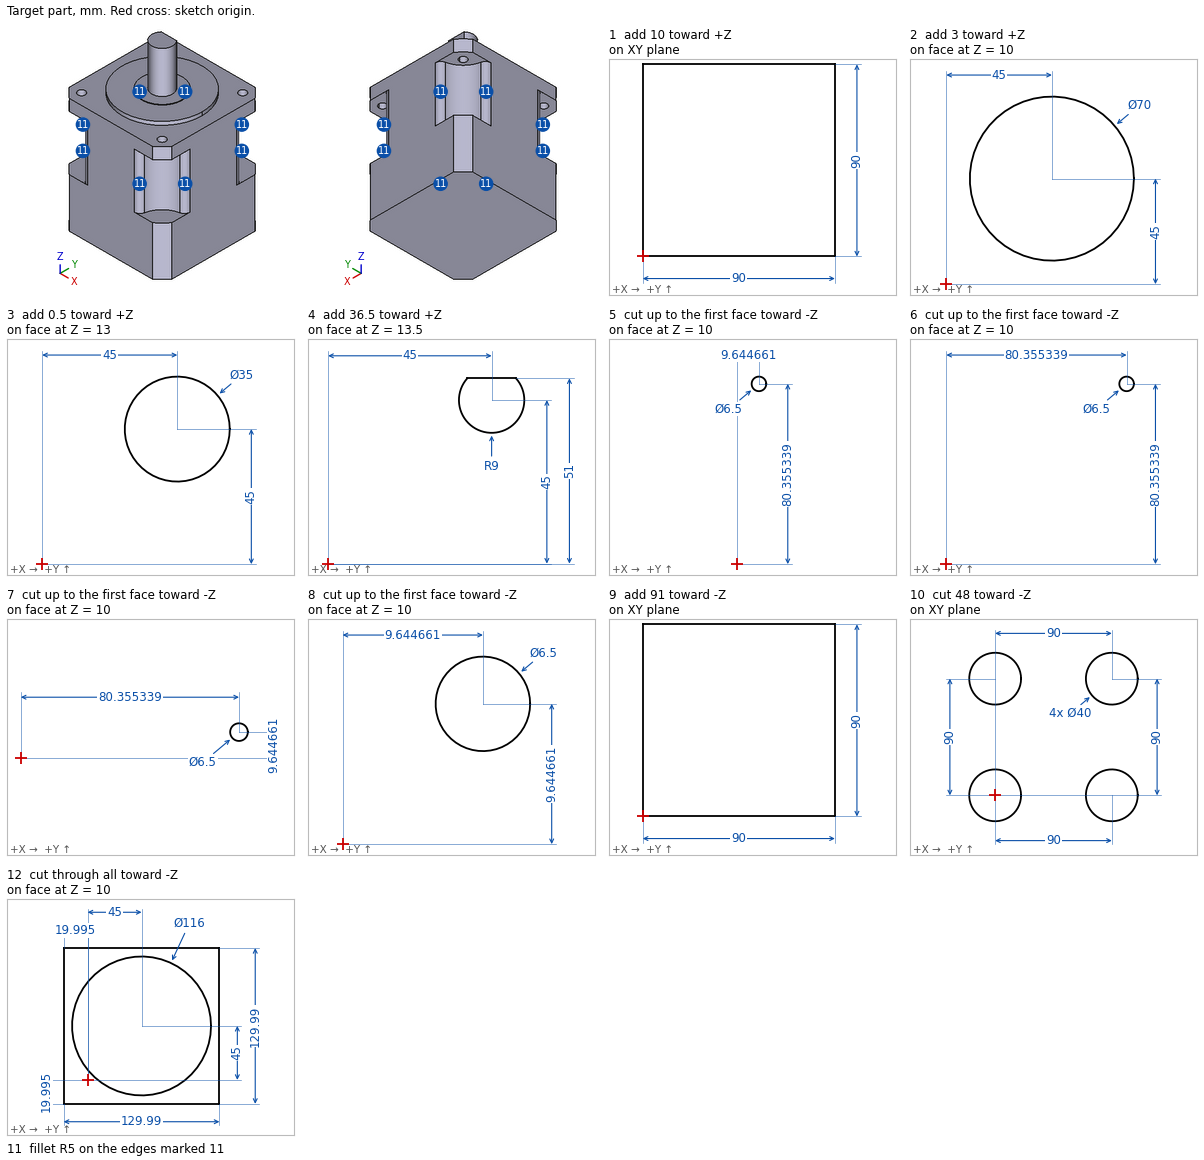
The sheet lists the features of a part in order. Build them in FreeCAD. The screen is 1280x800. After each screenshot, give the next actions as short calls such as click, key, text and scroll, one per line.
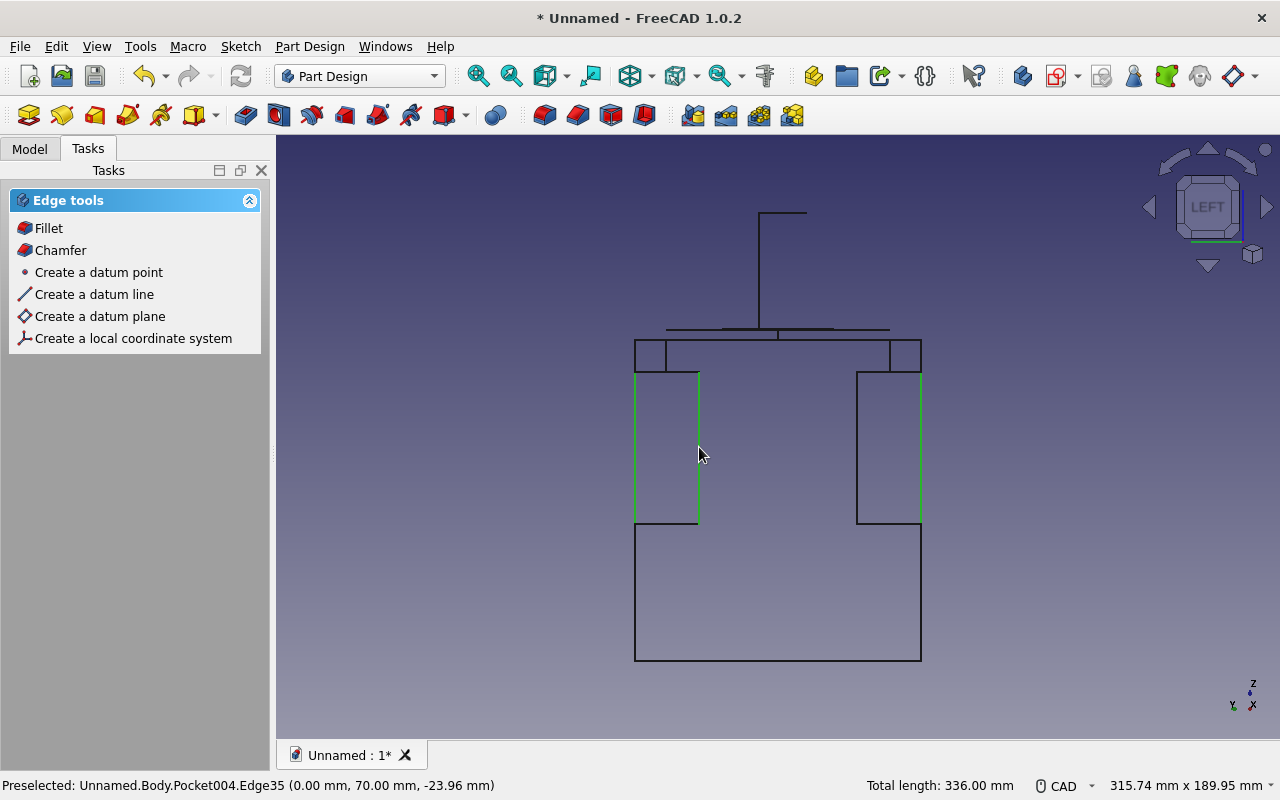
key(0)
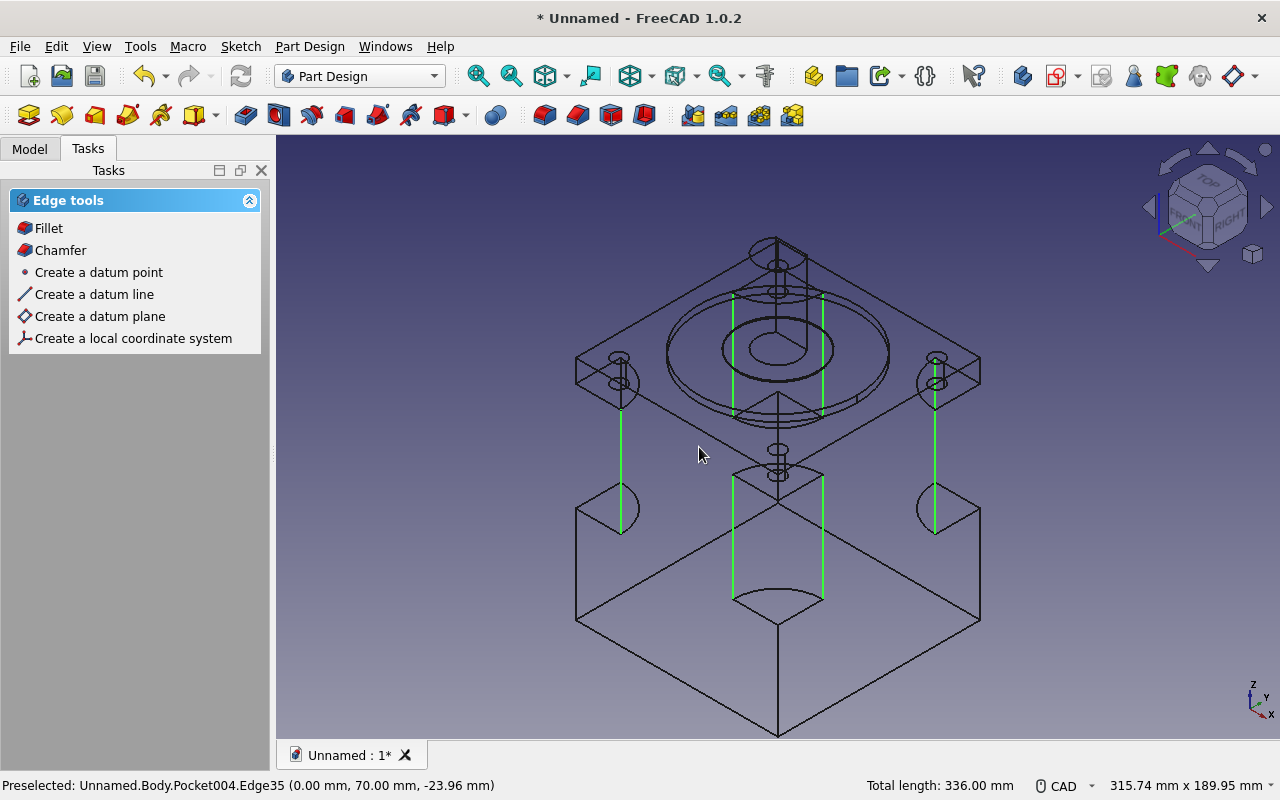
key(2)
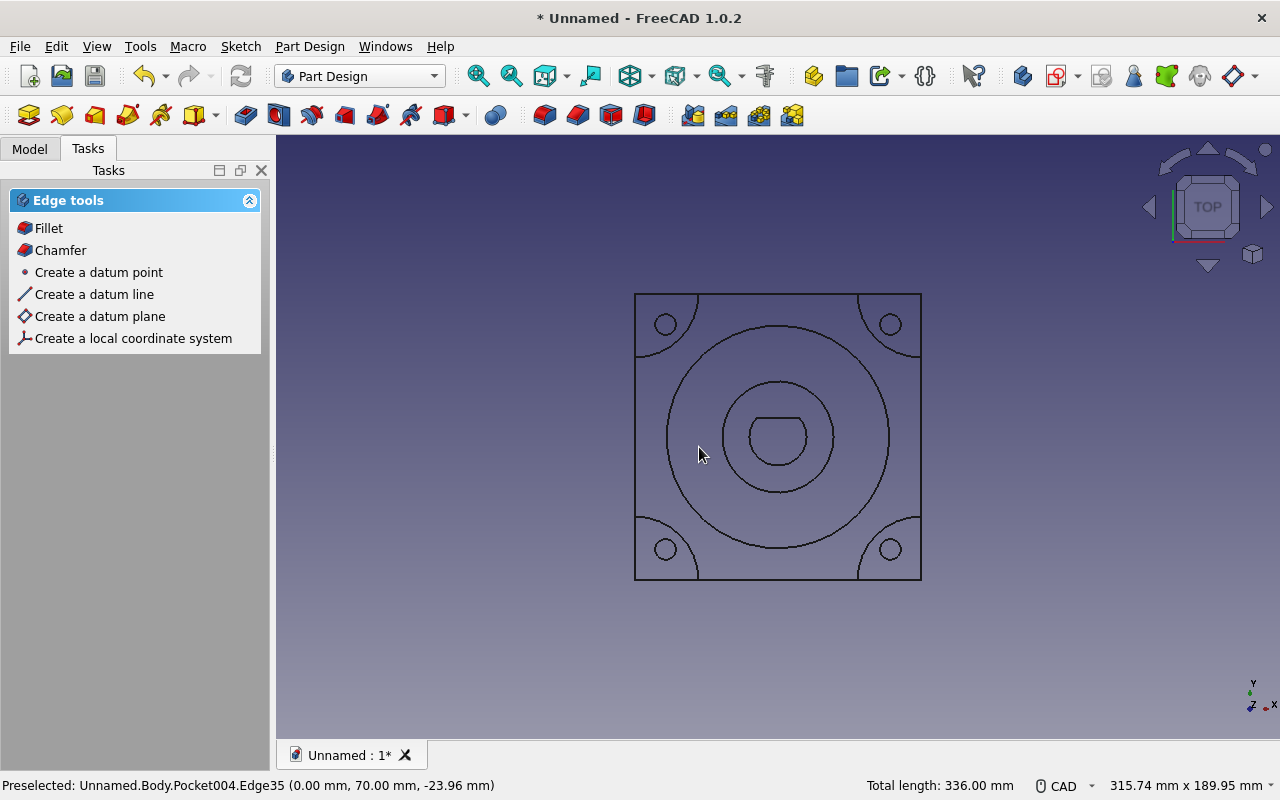
key(1)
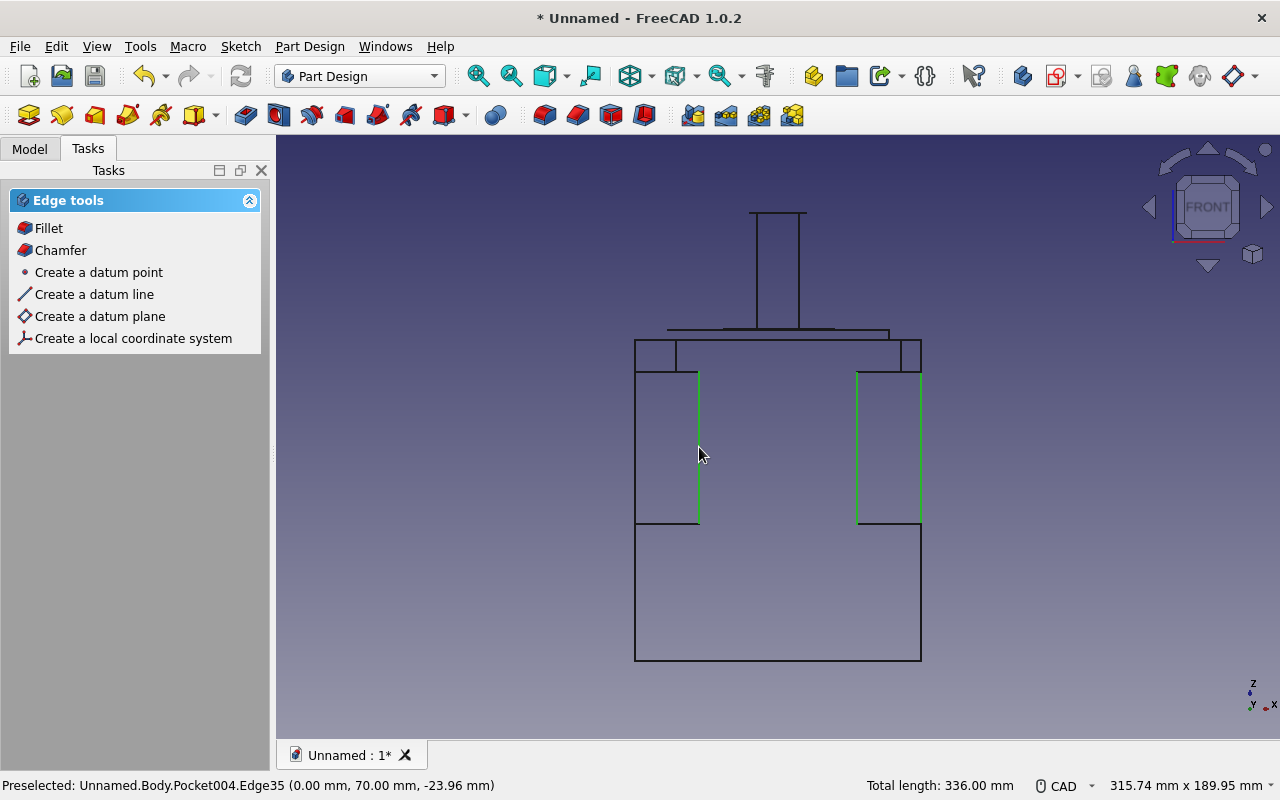
click(635, 447, ctrl)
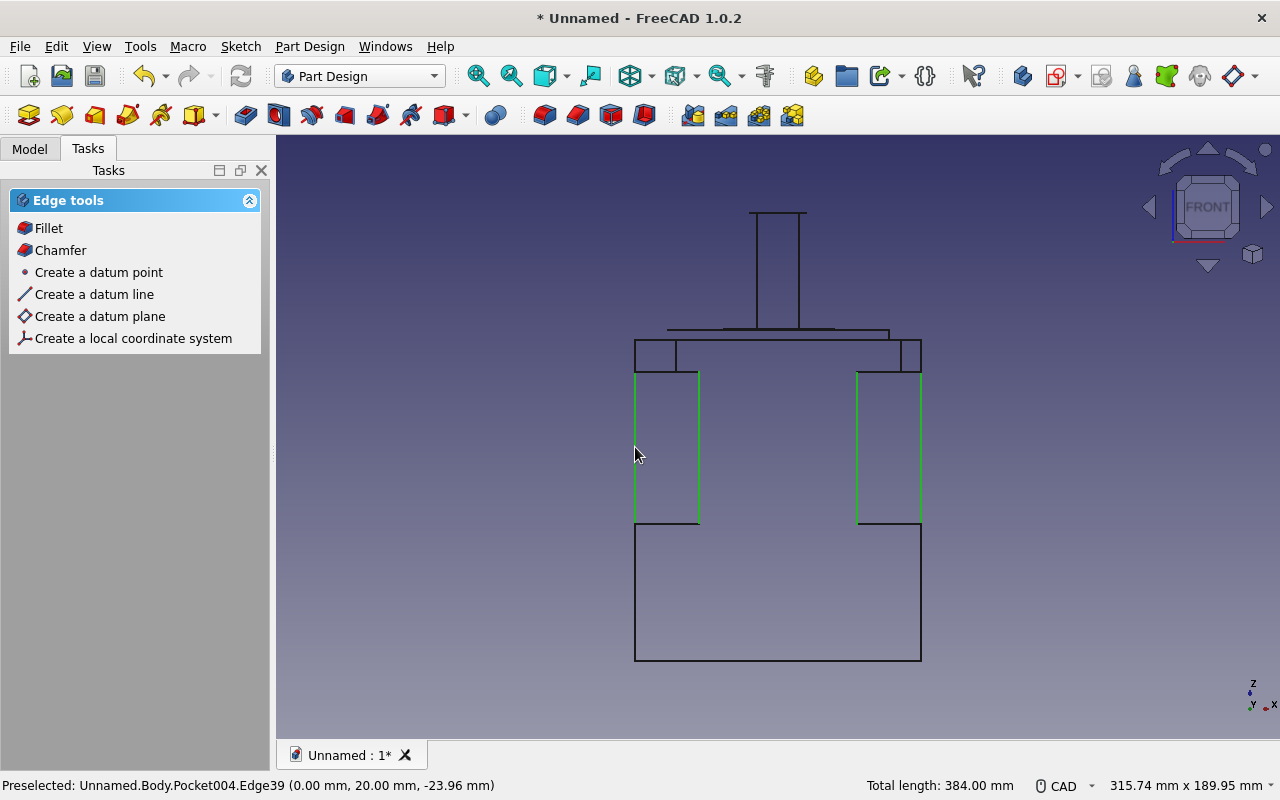
key(v)
key(1)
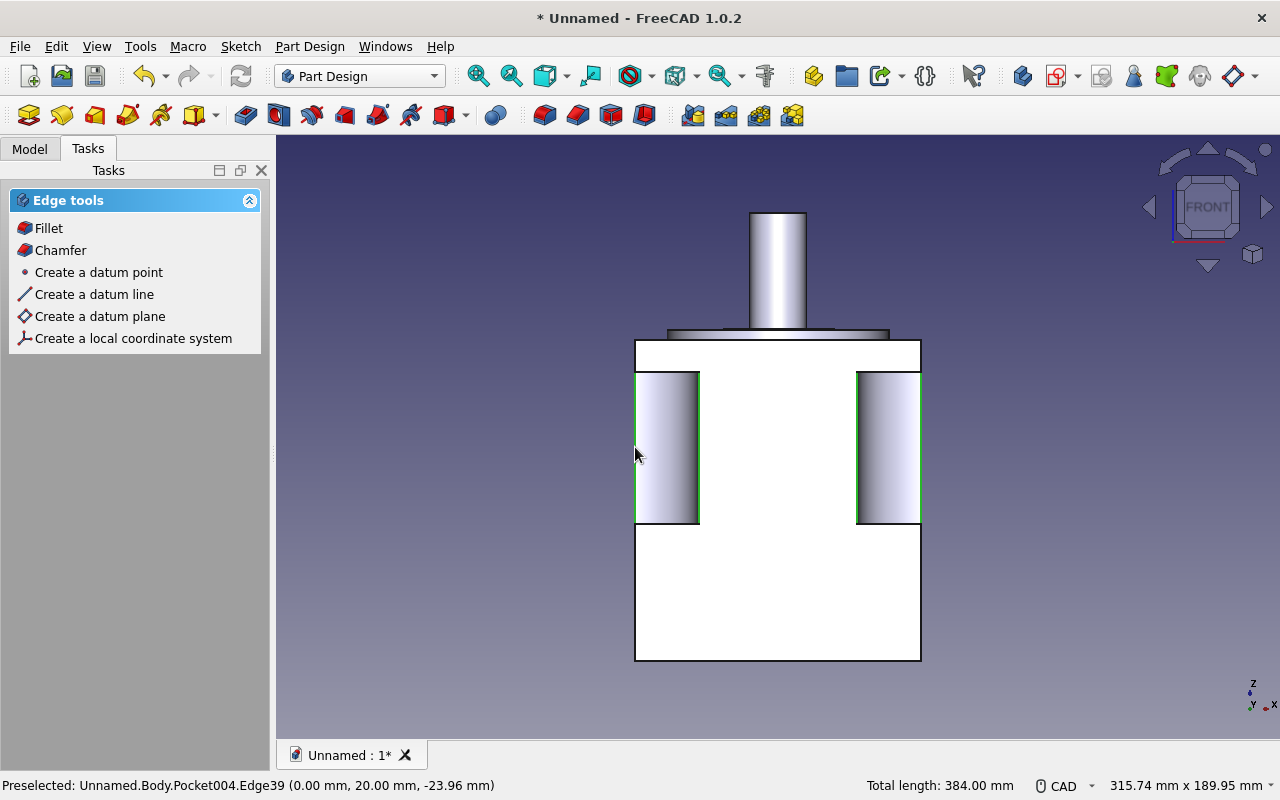
click(545, 116)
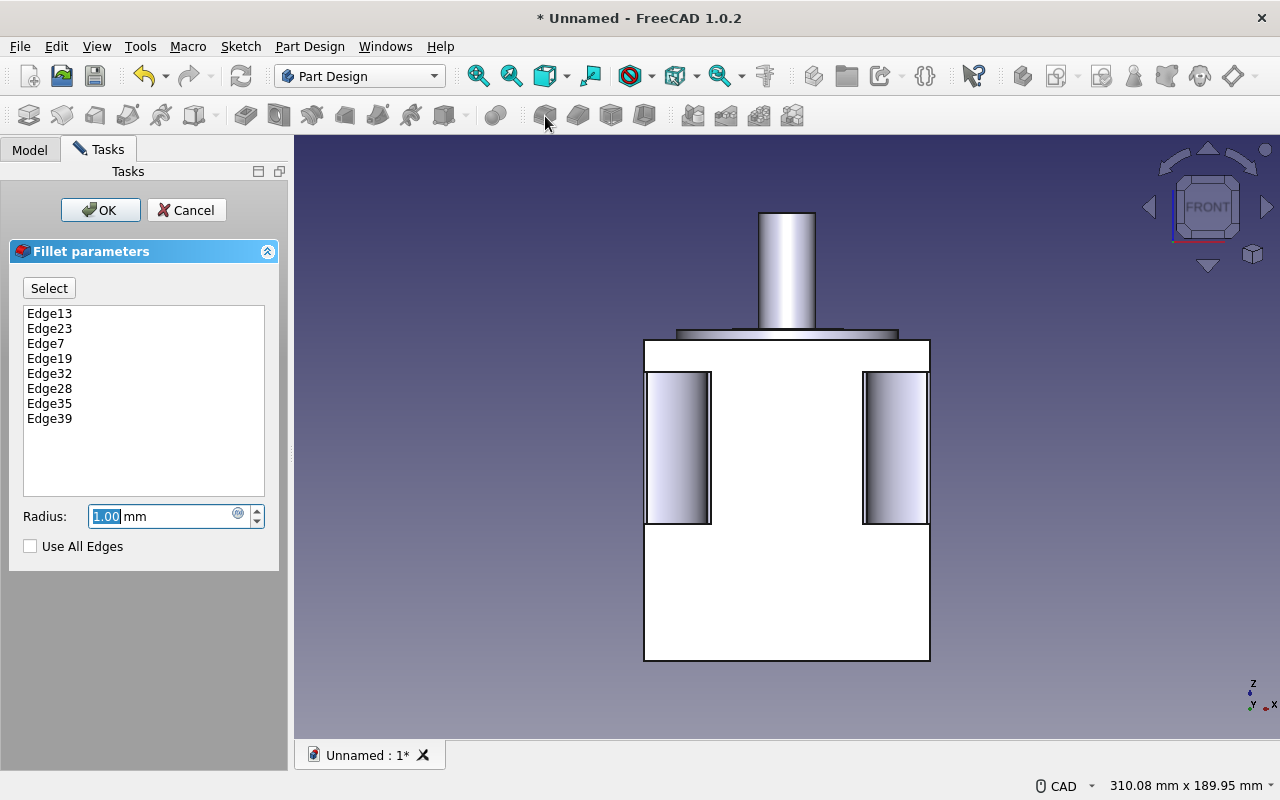
text(5)
key(Tab)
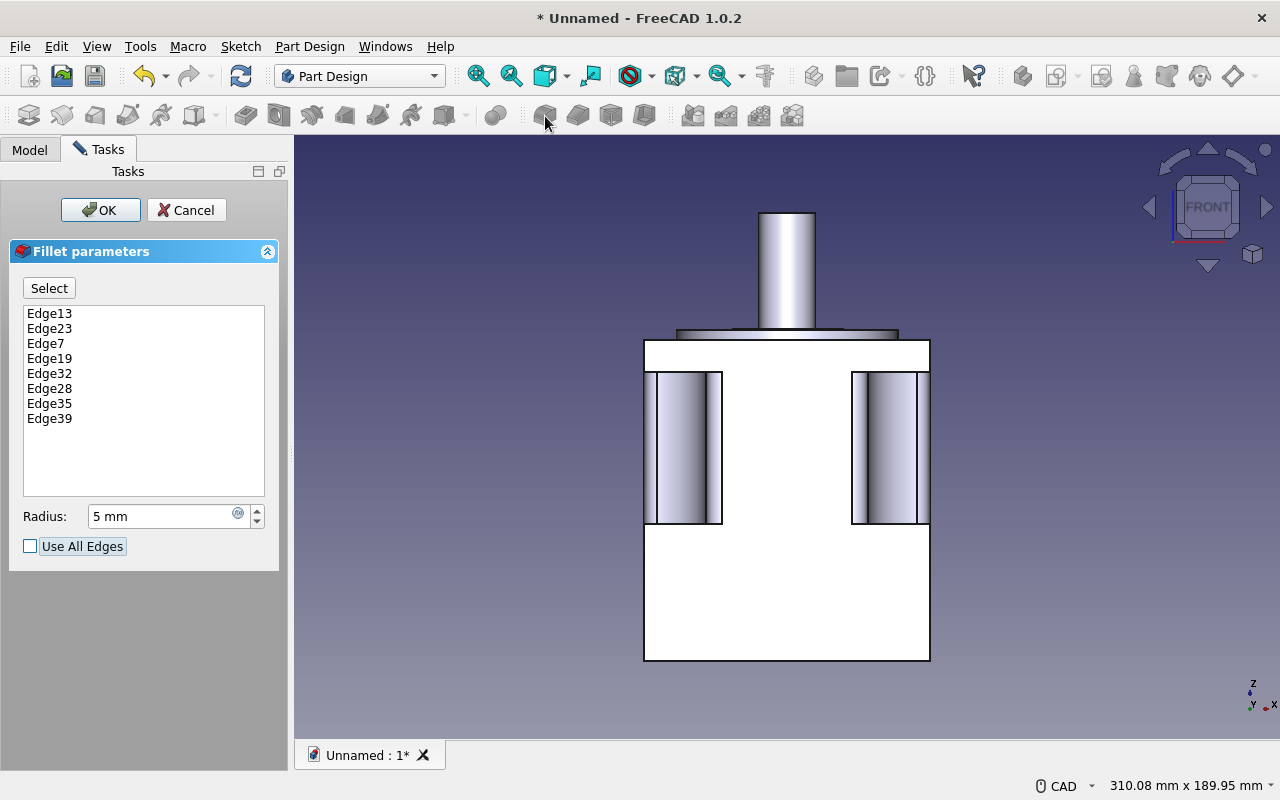
click(101, 210)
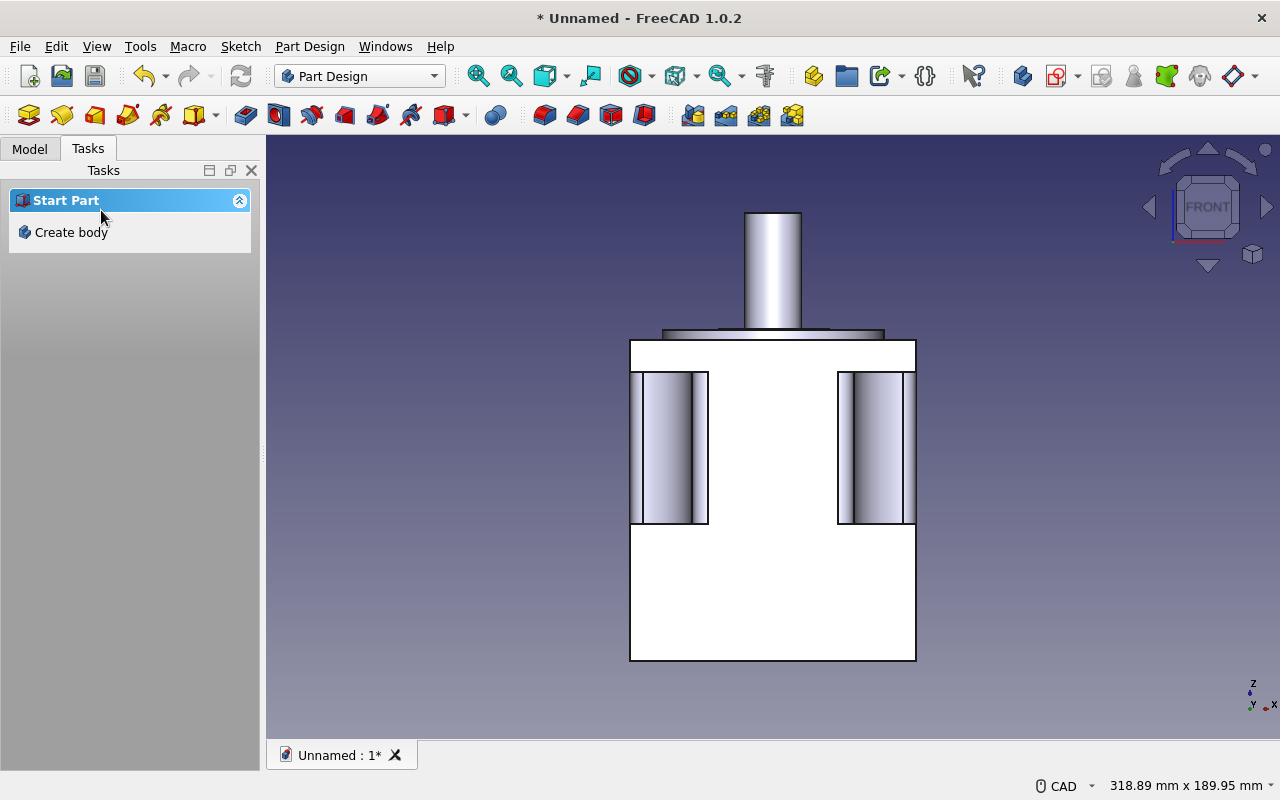
key(0)